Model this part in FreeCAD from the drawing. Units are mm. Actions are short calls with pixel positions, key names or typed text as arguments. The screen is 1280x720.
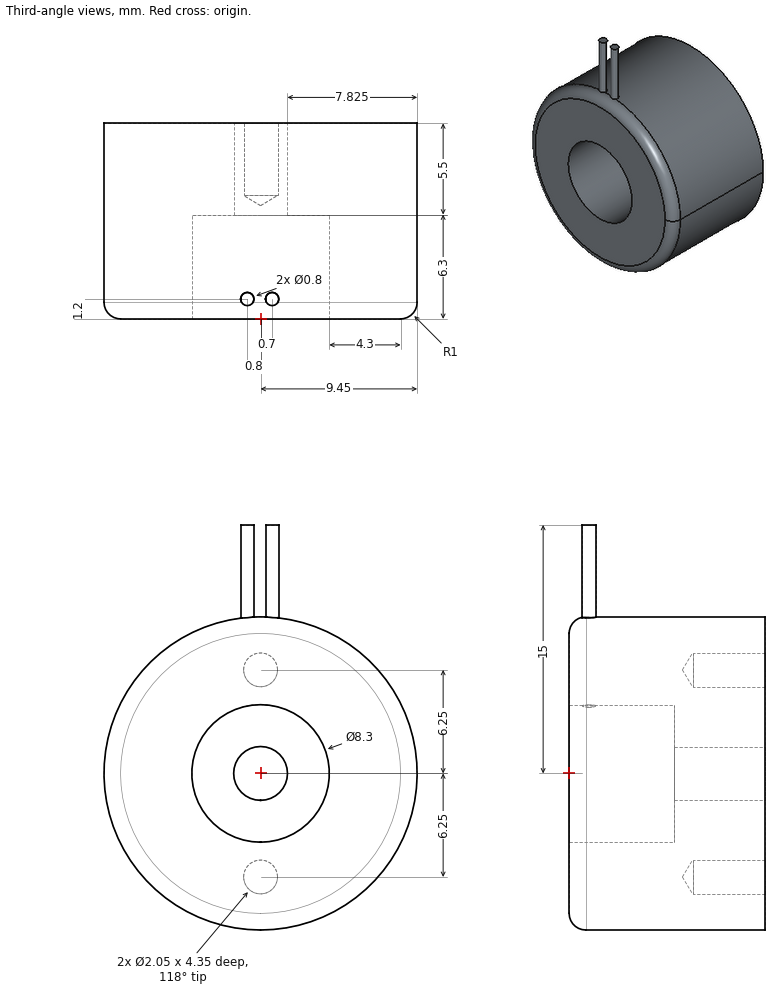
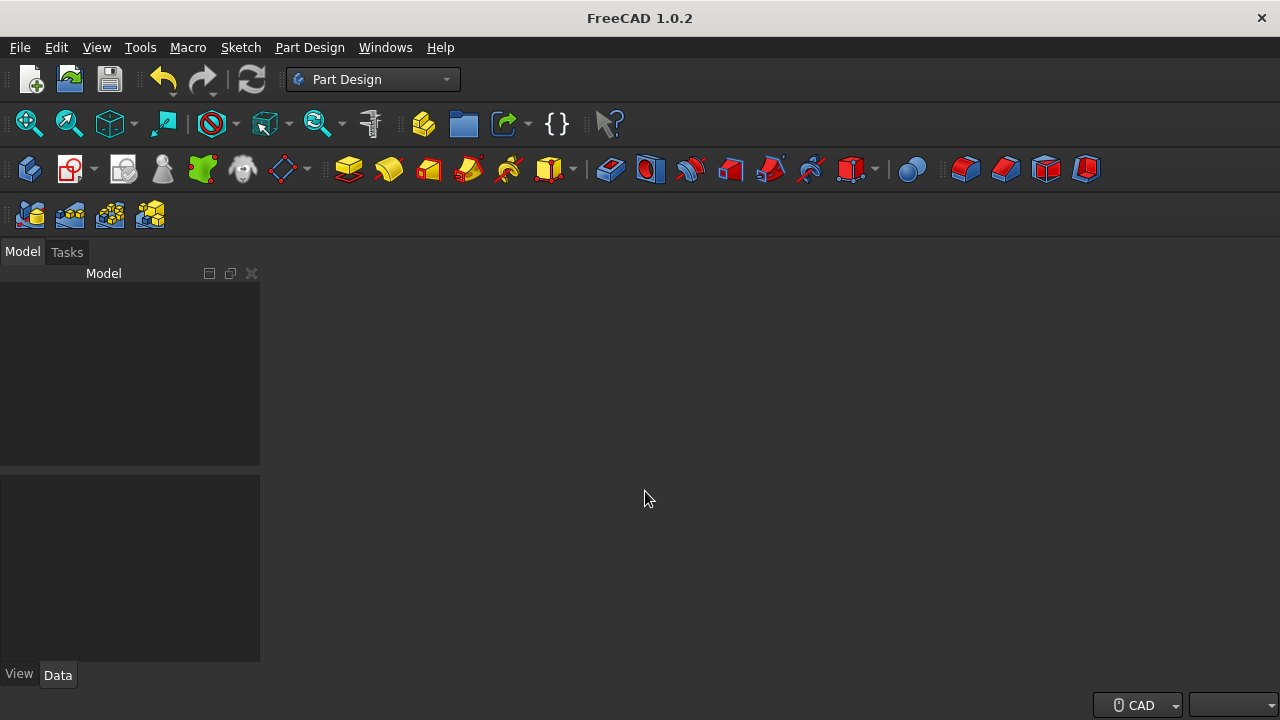
key(ctrl+n)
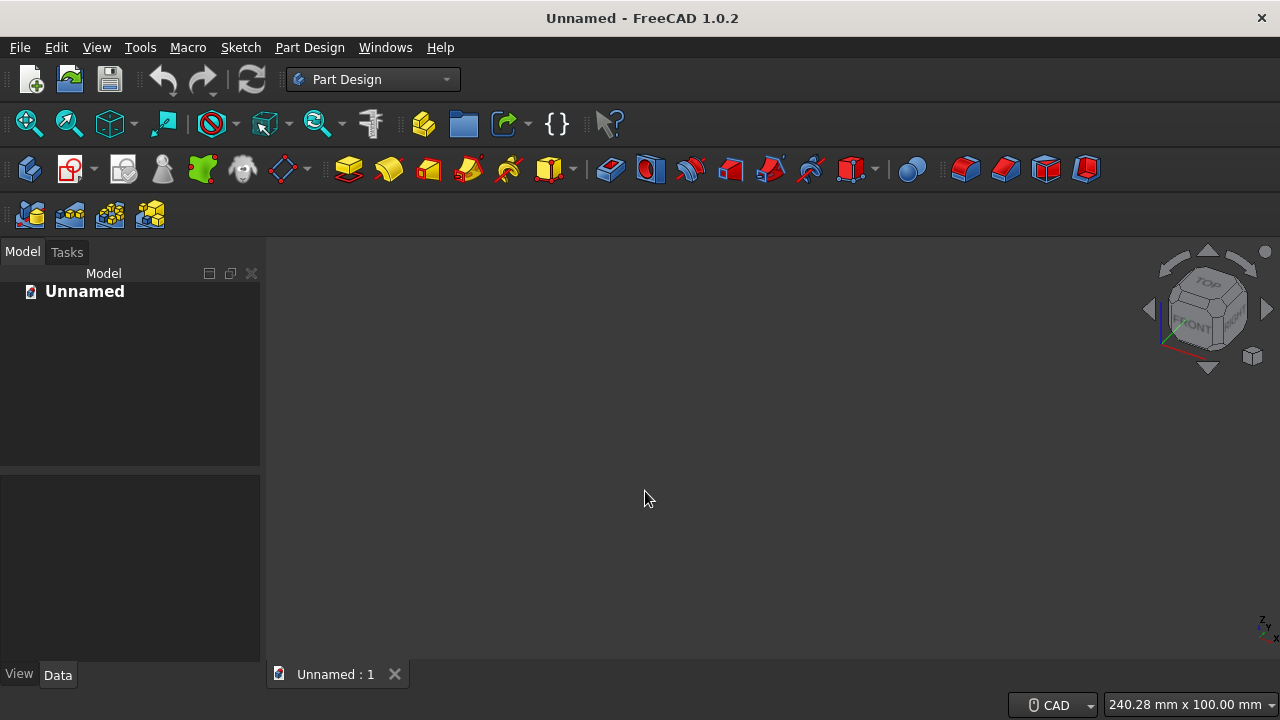
click(70, 170)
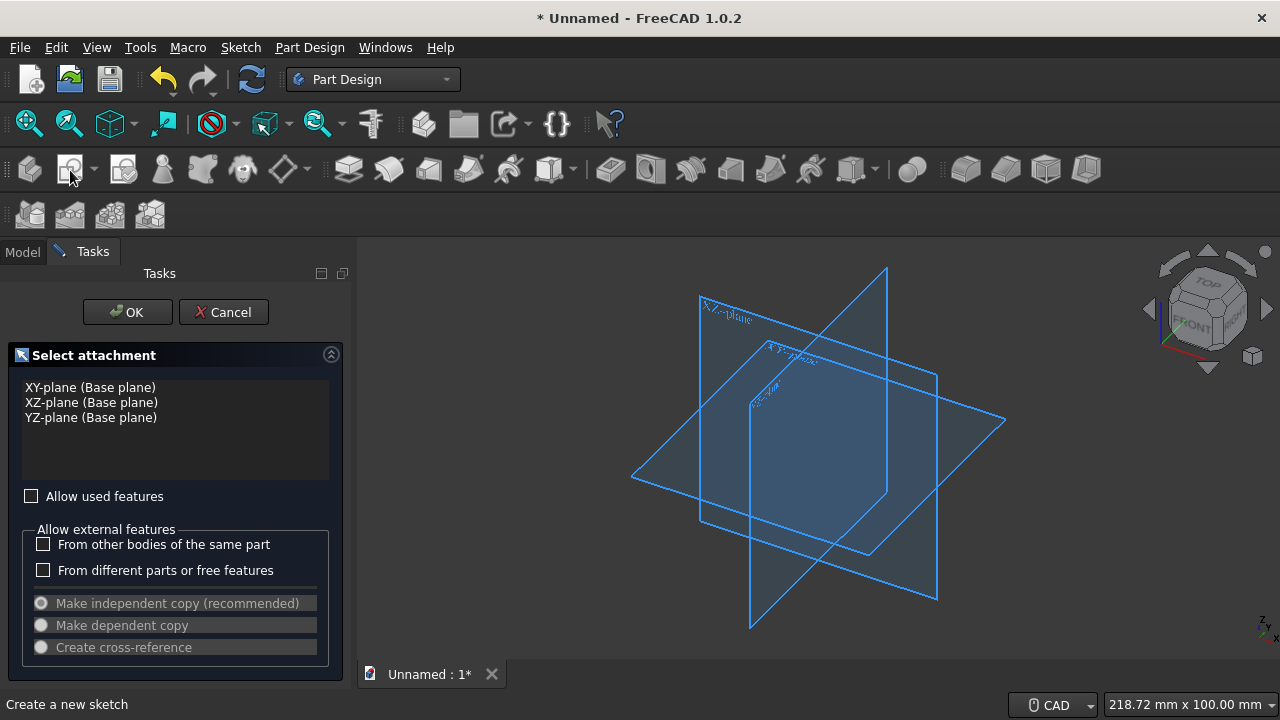
click(82, 388)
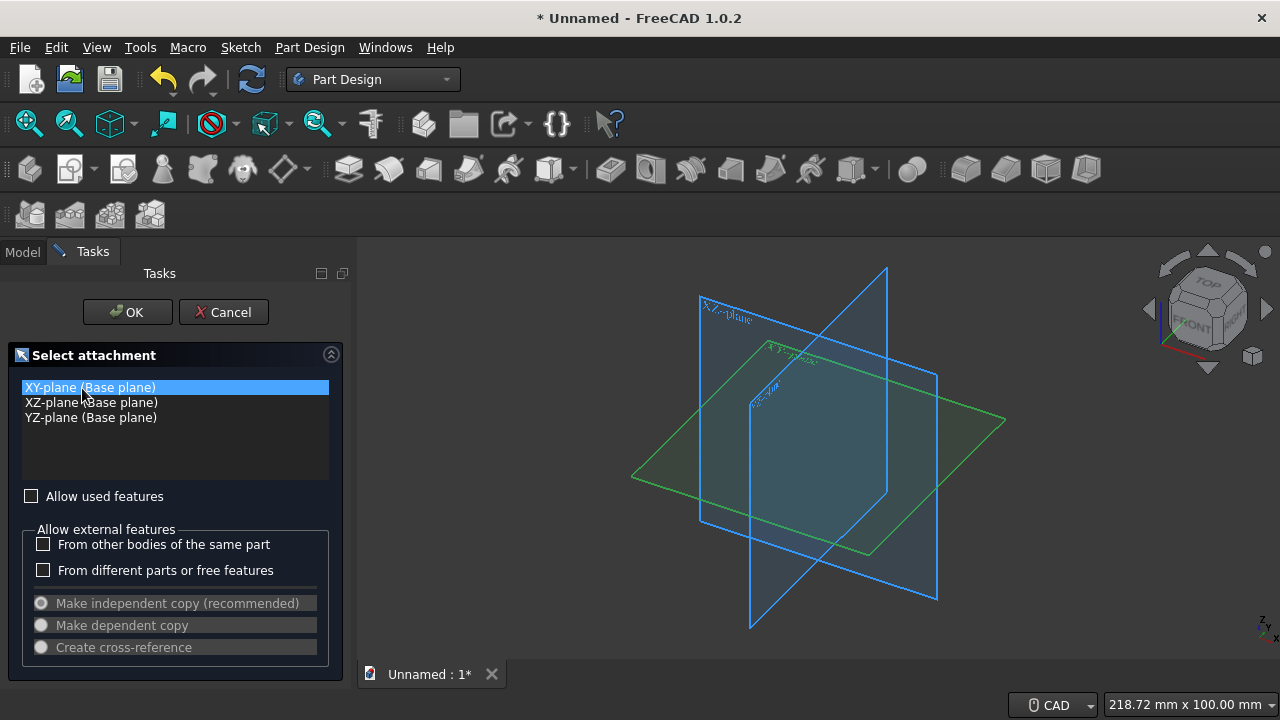
click(128, 312)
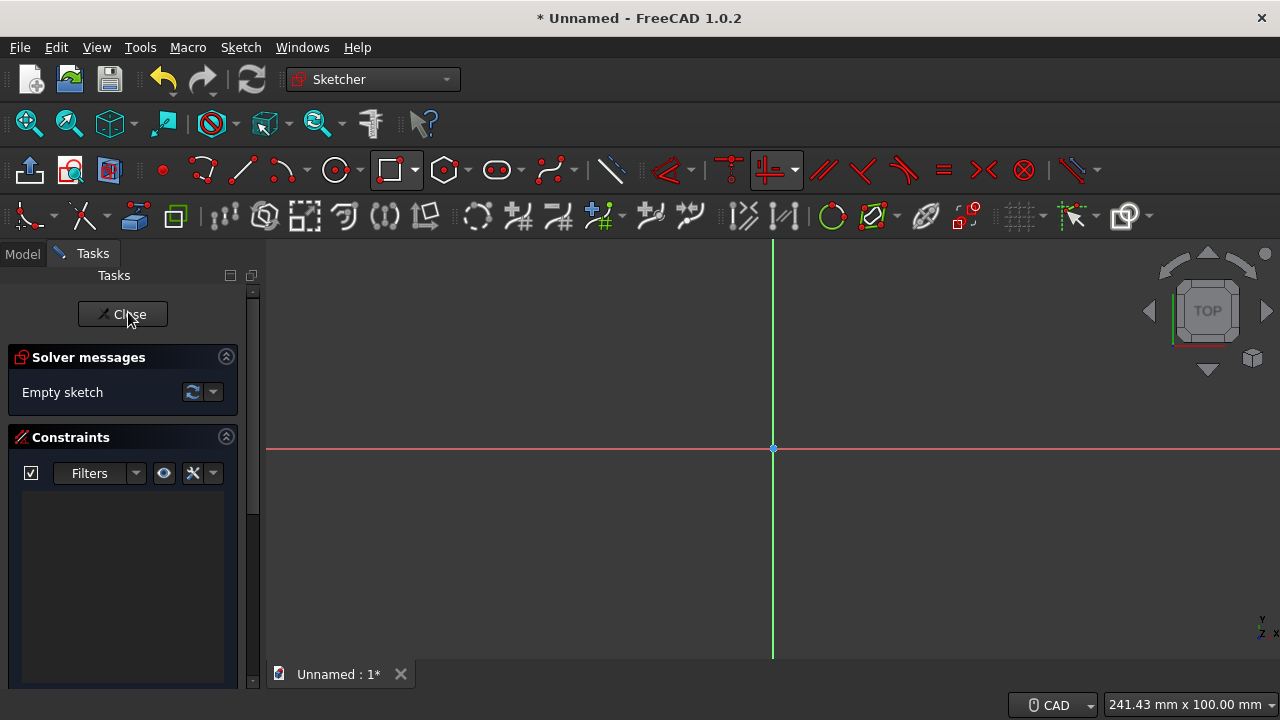
scroll(815, 418, up, 8)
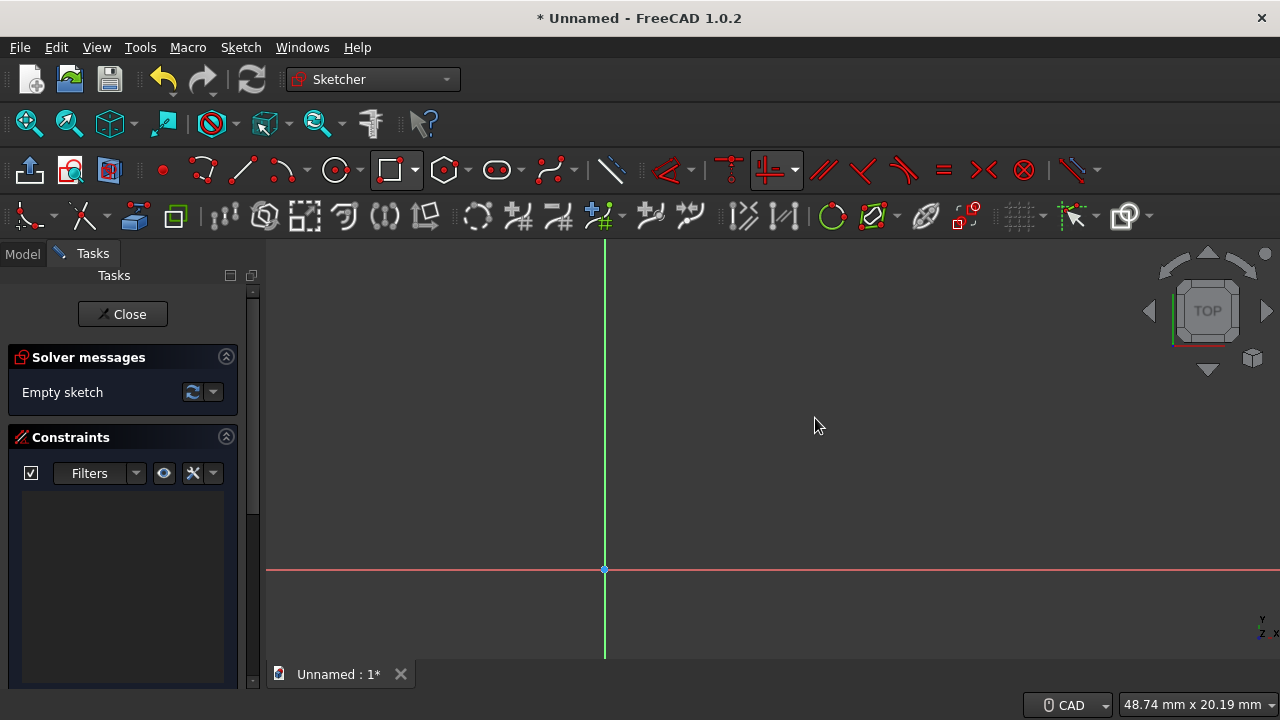
click(204, 170)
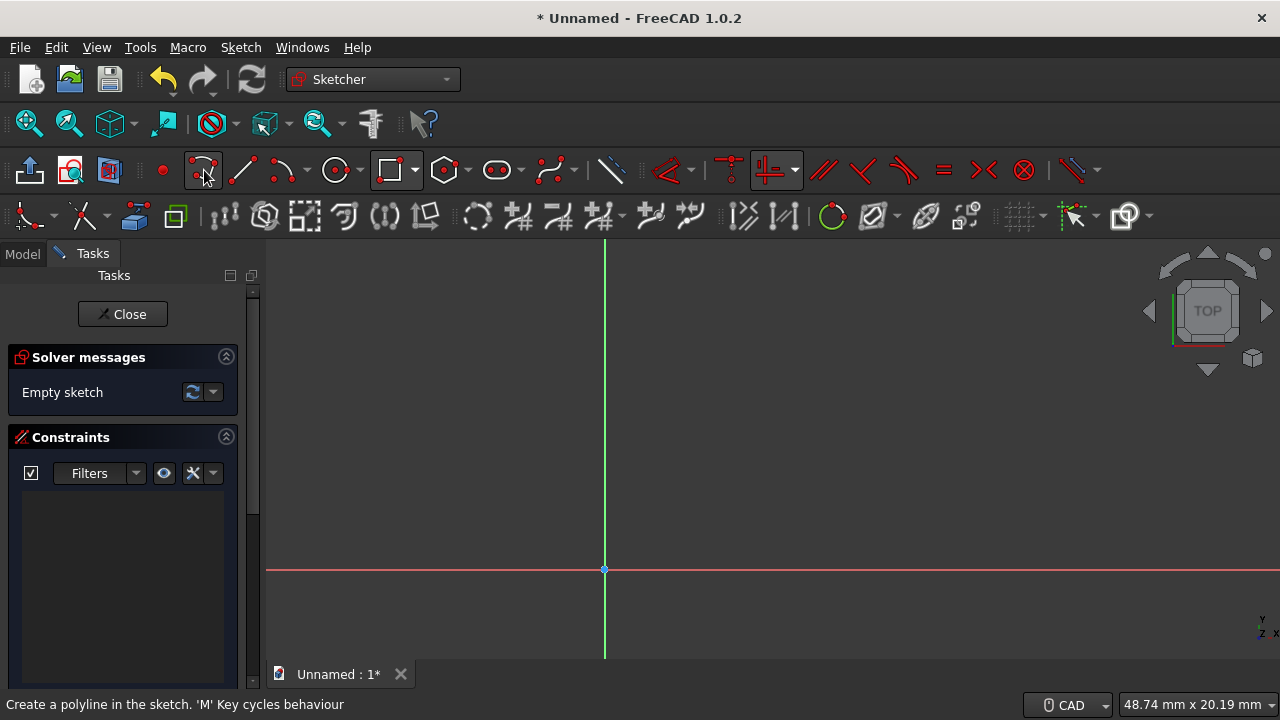
click(801, 549)
click(801, 324)
click(639, 324)
click(639, 439)
click(691, 439)
click(691, 570)
click(781, 561)
right_click(781, 561)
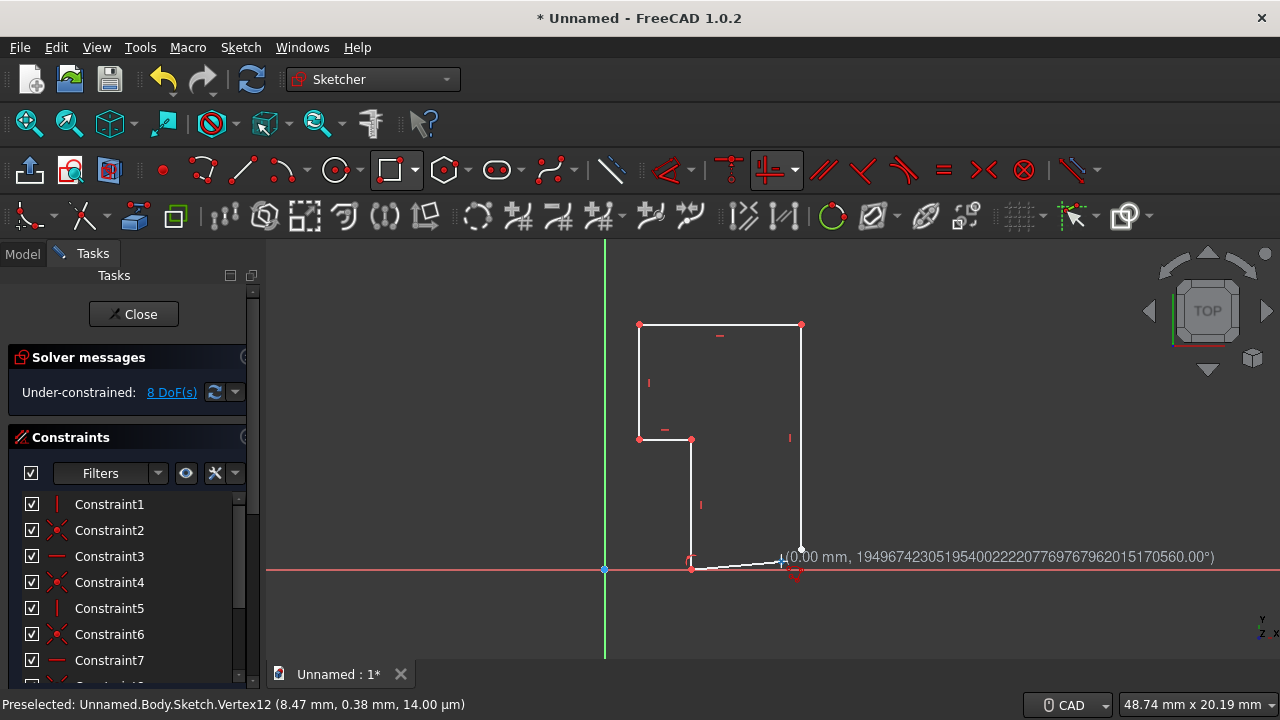
key(g)
key(3)
key(a)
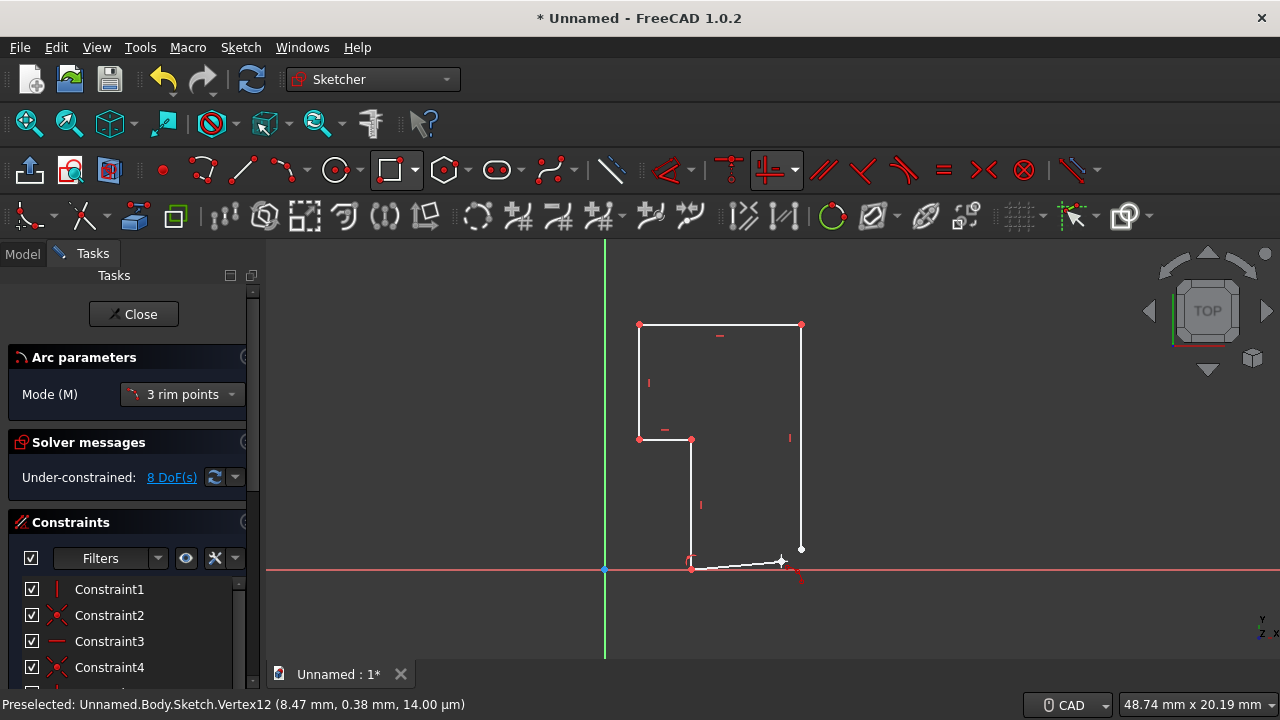
click(781, 562)
click(801, 550)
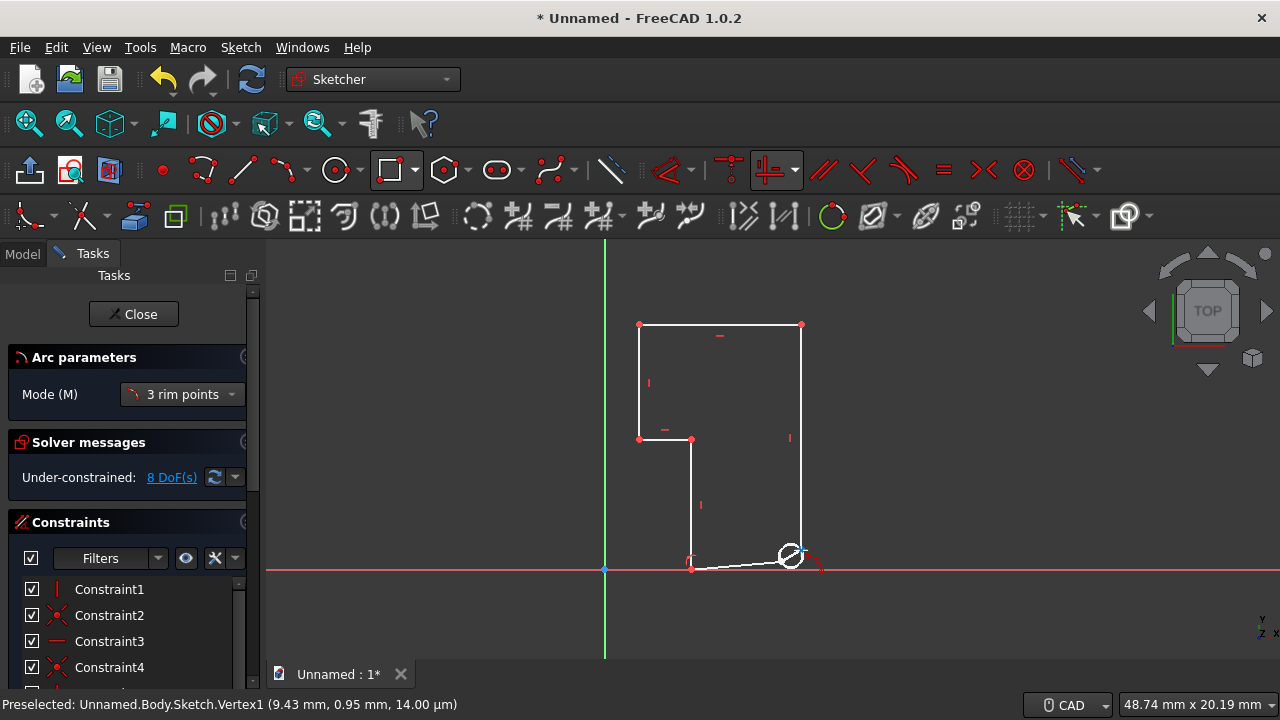
scroll(795, 564, up, 5)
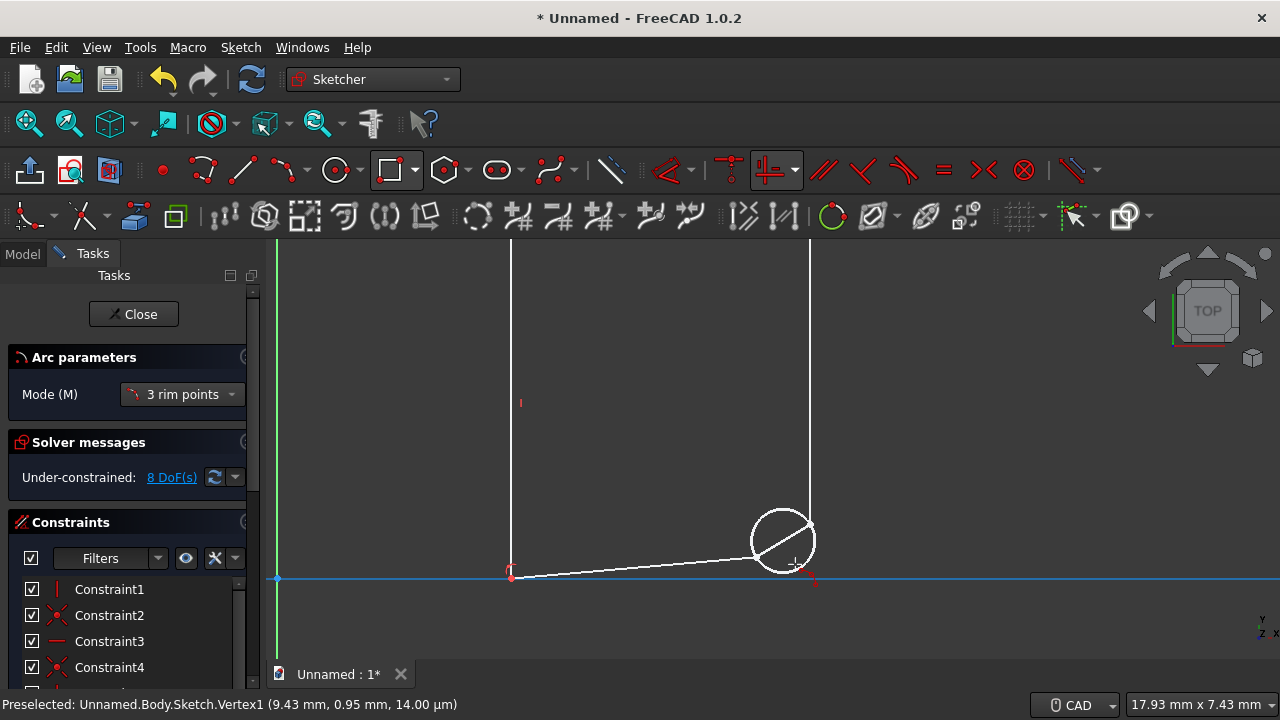
click(795, 562)
key(Escape)